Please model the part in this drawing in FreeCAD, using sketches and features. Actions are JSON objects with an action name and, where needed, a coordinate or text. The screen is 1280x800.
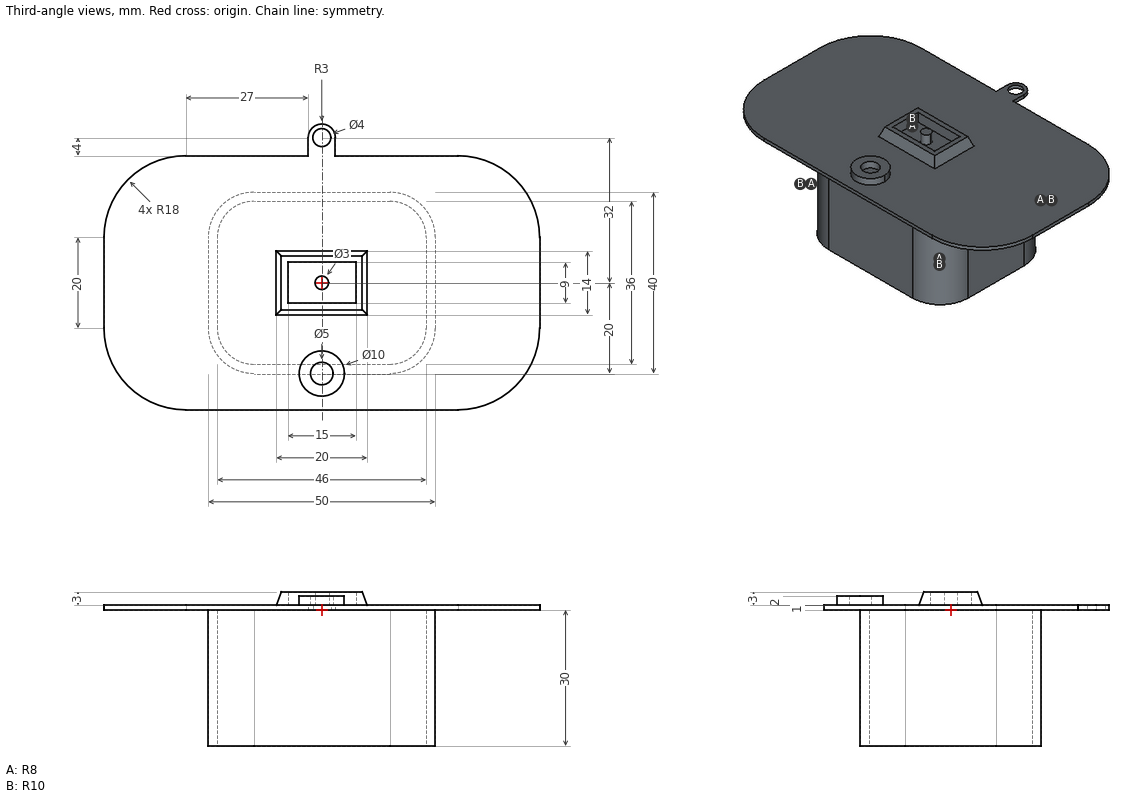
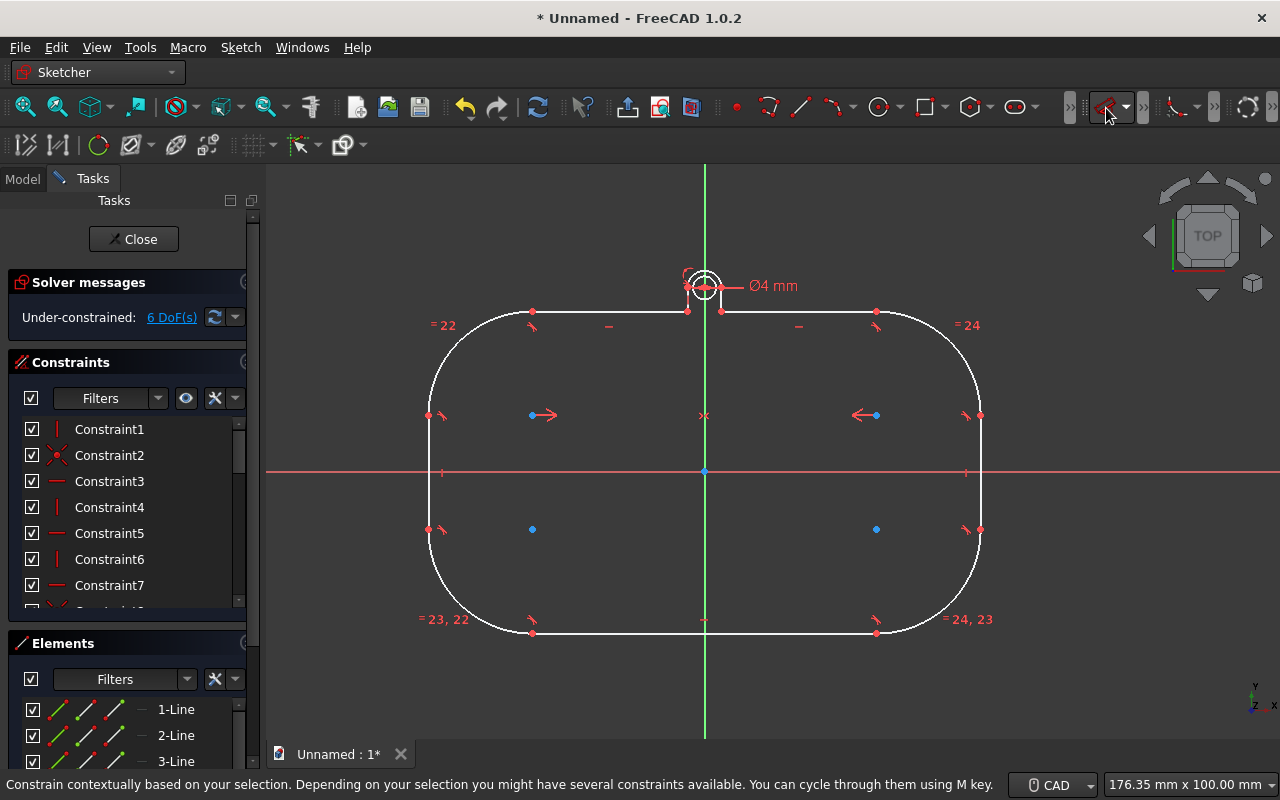
{"action": "left_click", "coordinate": [485, 323]}
{"action": "left_click", "coordinate": [470, 295]}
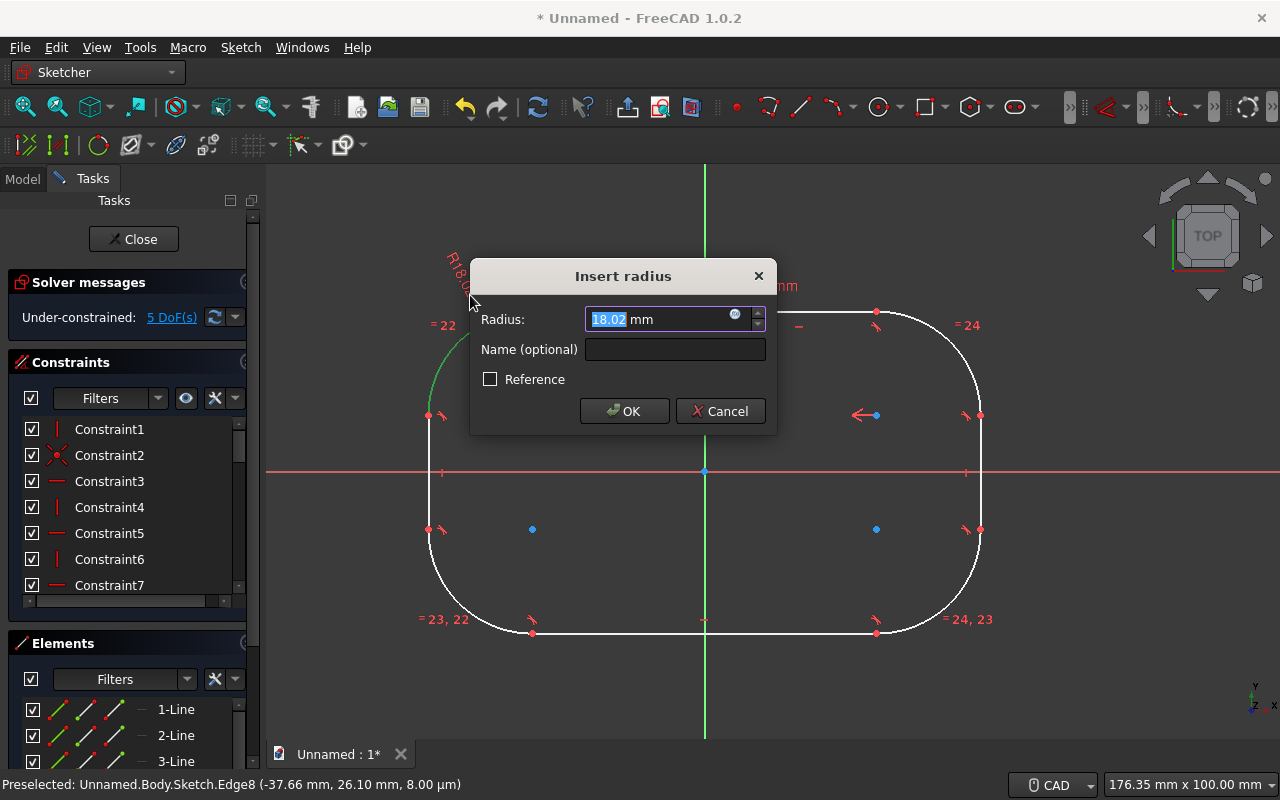
{"action": "type", "text": "18"}
{"action": "key", "text": "Return"}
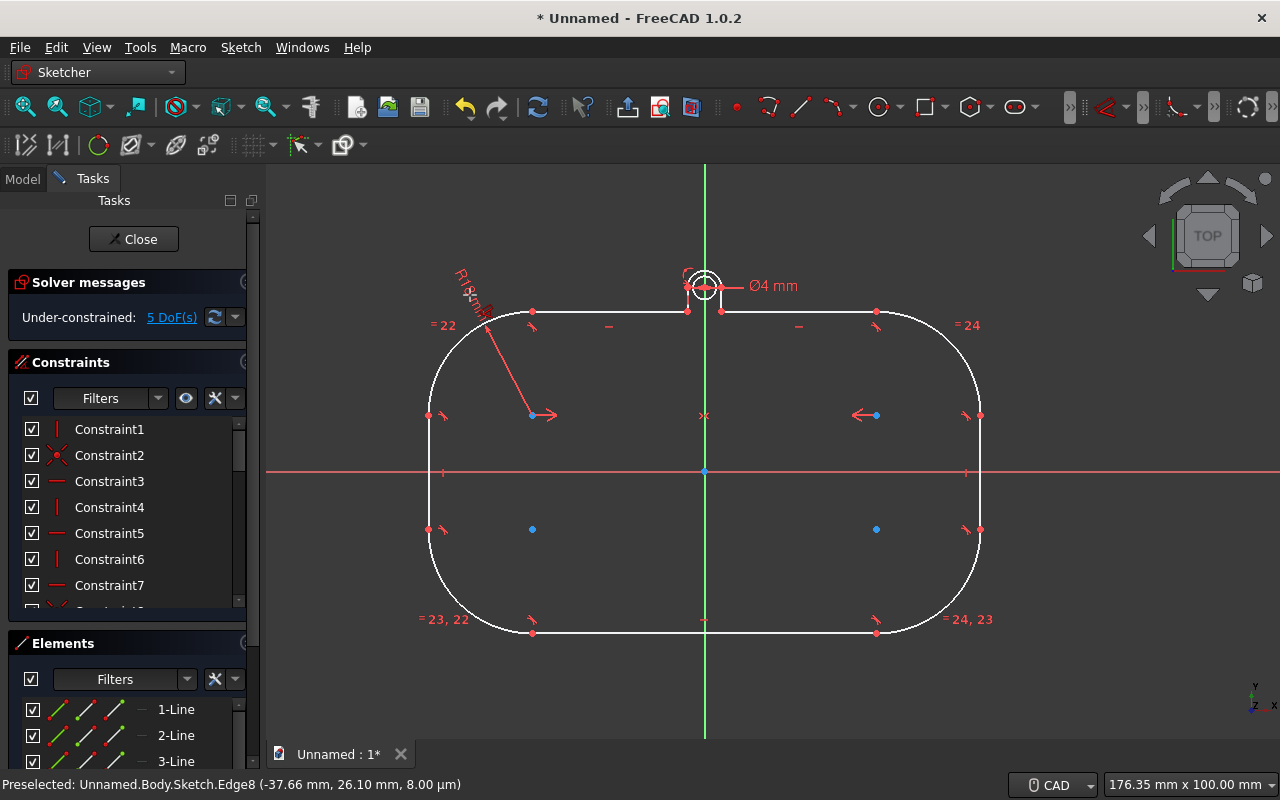
{"action": "scroll", "coordinate": [718, 278], "scroll_direction": "up", "scroll_amount": 5}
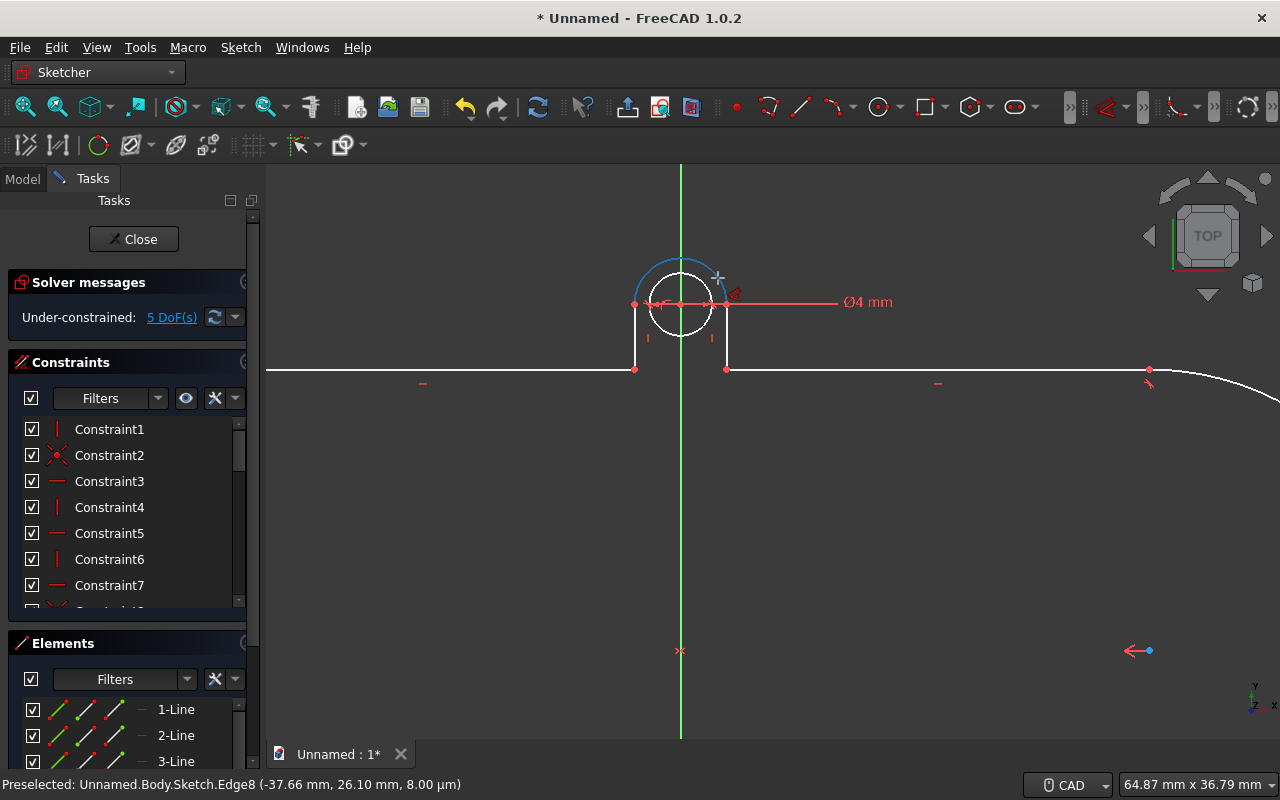
{"action": "left_click", "coordinate": [718, 277]}
{"action": "left_click", "coordinate": [744, 258]}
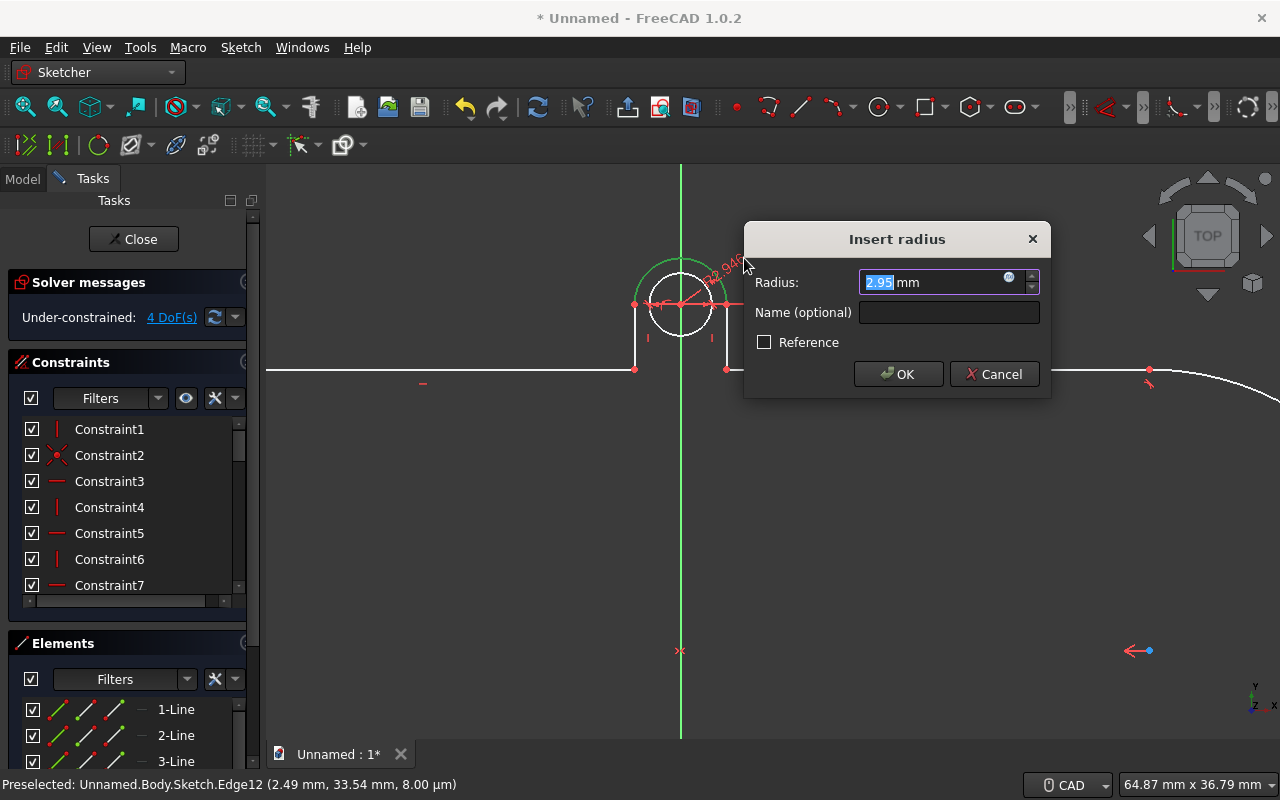
{"action": "type", "text": "3"}
{"action": "key", "text": "Return"}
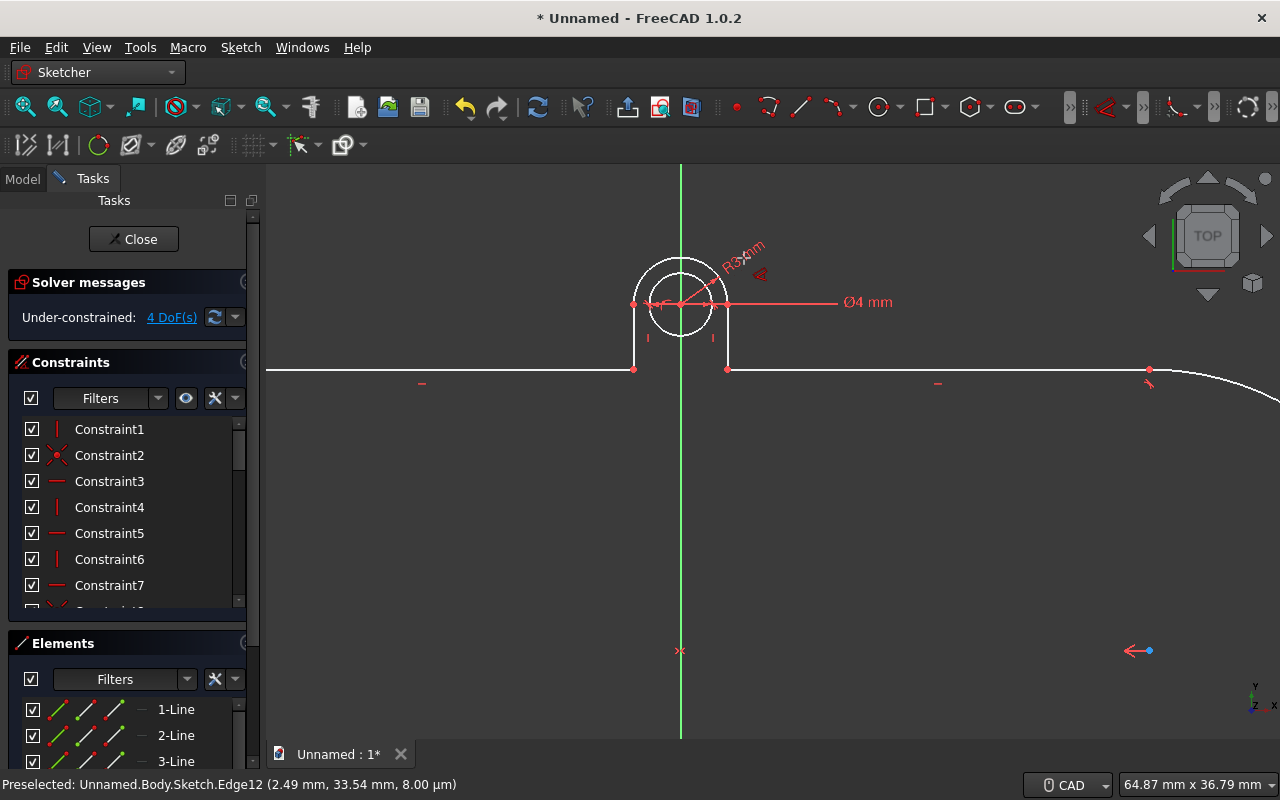
{"action": "left_click", "coordinate": [634, 324]}
{"action": "left_click", "coordinate": [600, 337]}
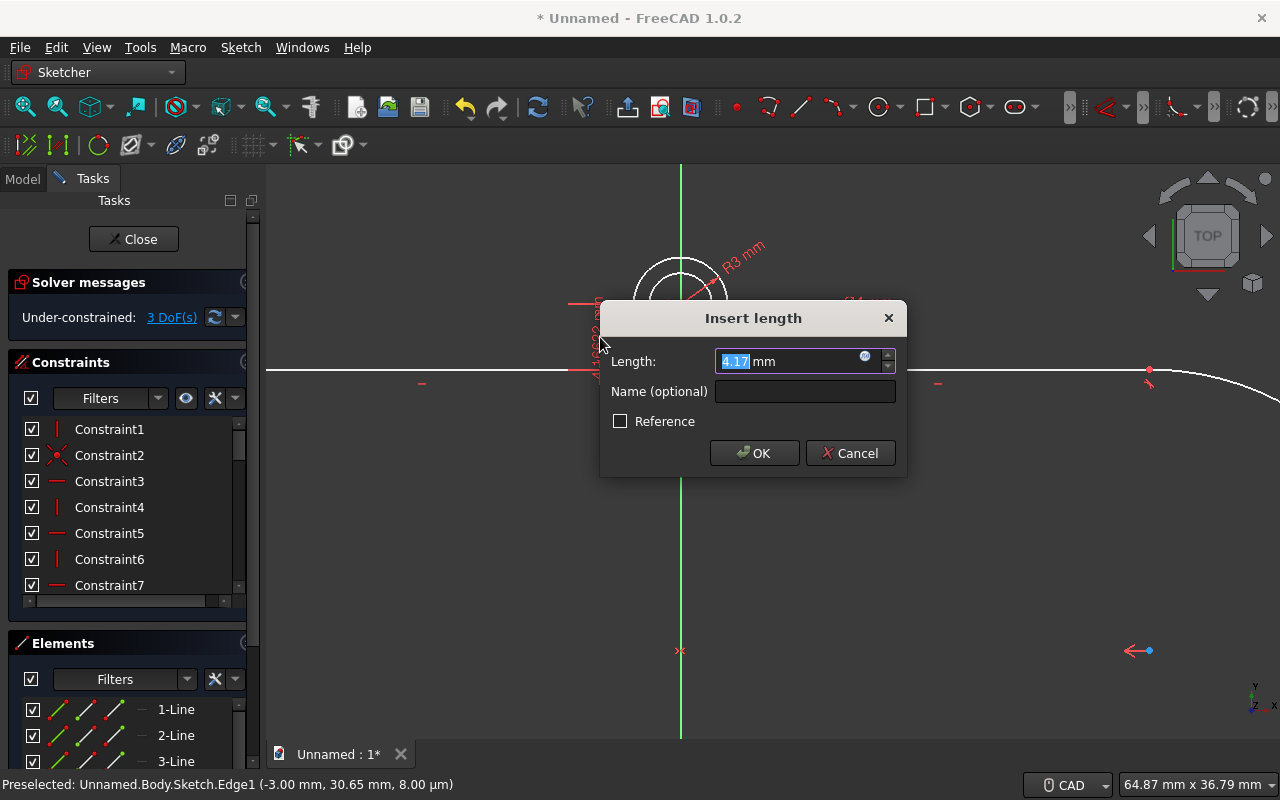
{"action": "type", "text": "4"}
{"action": "key", "text": "Return"}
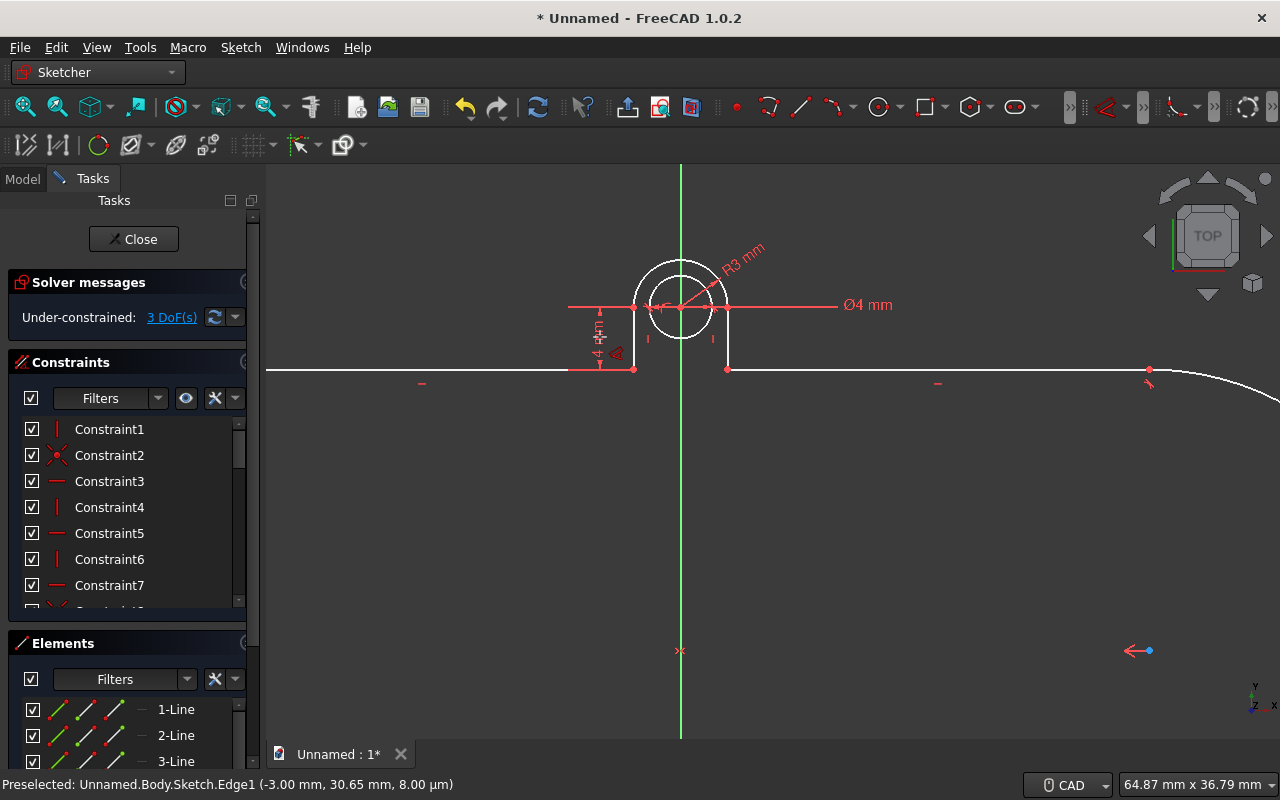
{"action": "left_click", "coordinate": [507, 370]}
{"action": "left_click", "coordinate": [464, 336]}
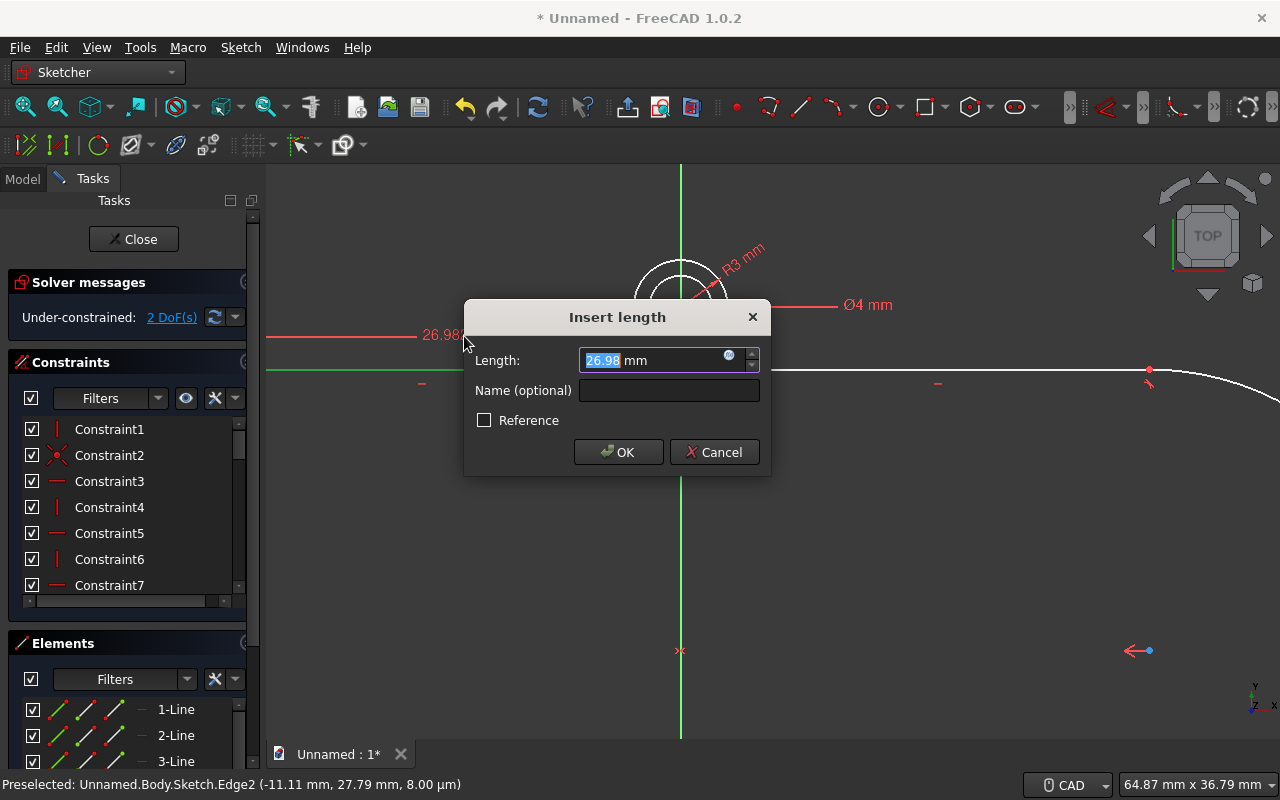
{"action": "type", "text": "27"}
{"action": "key", "text": "Return"}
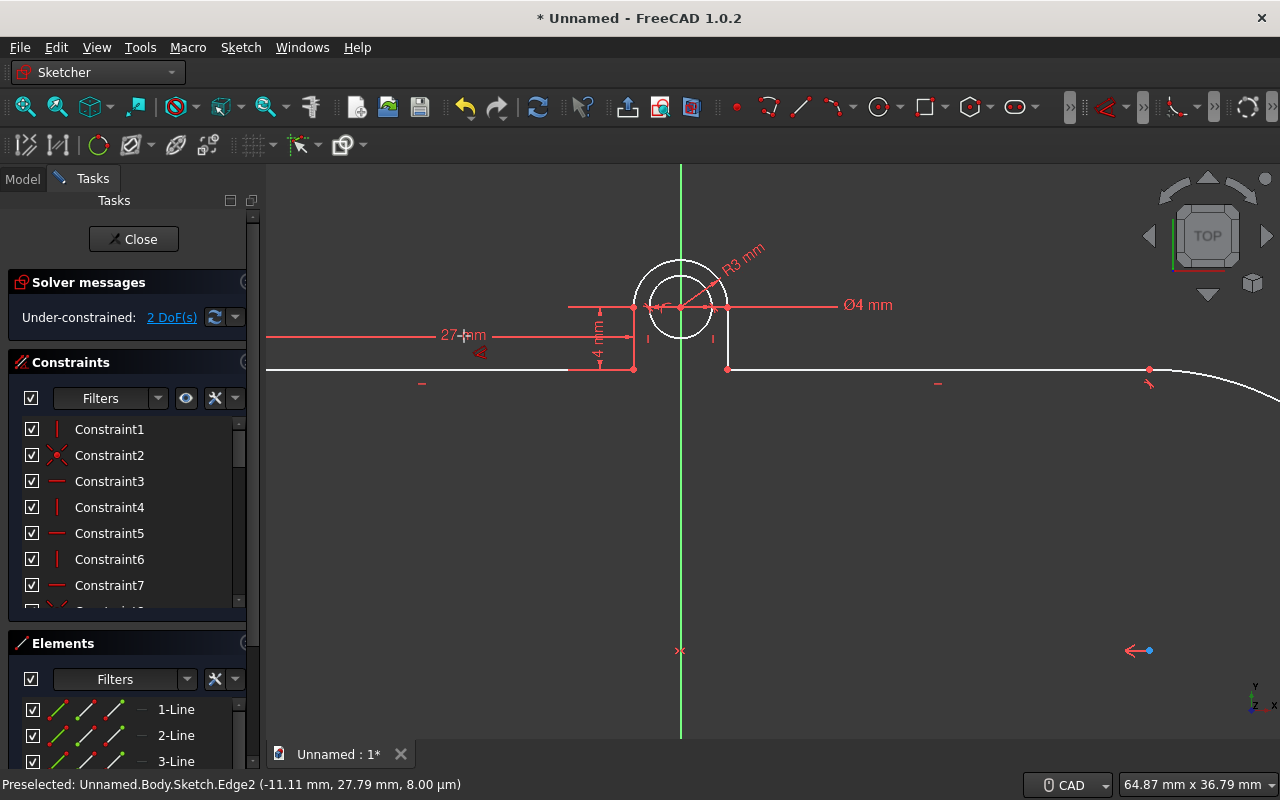
{"action": "scroll", "coordinate": [718, 278], "scroll_direction": "down", "scroll_amount": 5}